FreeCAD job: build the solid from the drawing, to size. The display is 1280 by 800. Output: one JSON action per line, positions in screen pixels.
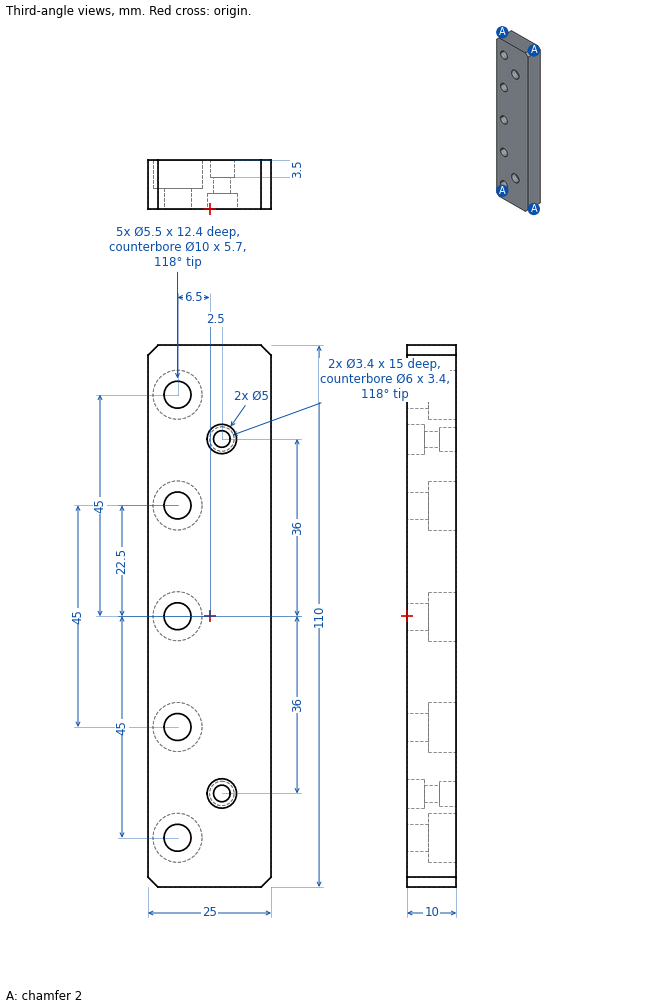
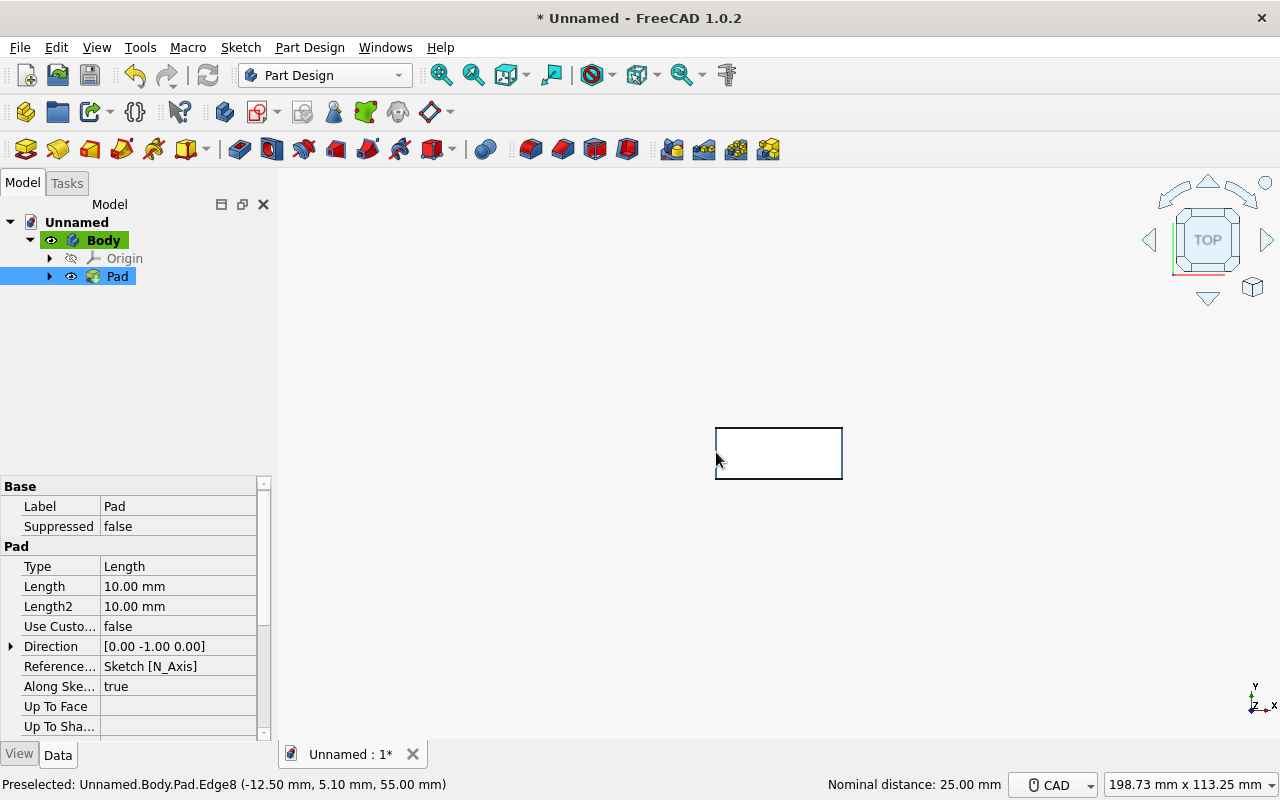
{"action": "key", "text": "1"}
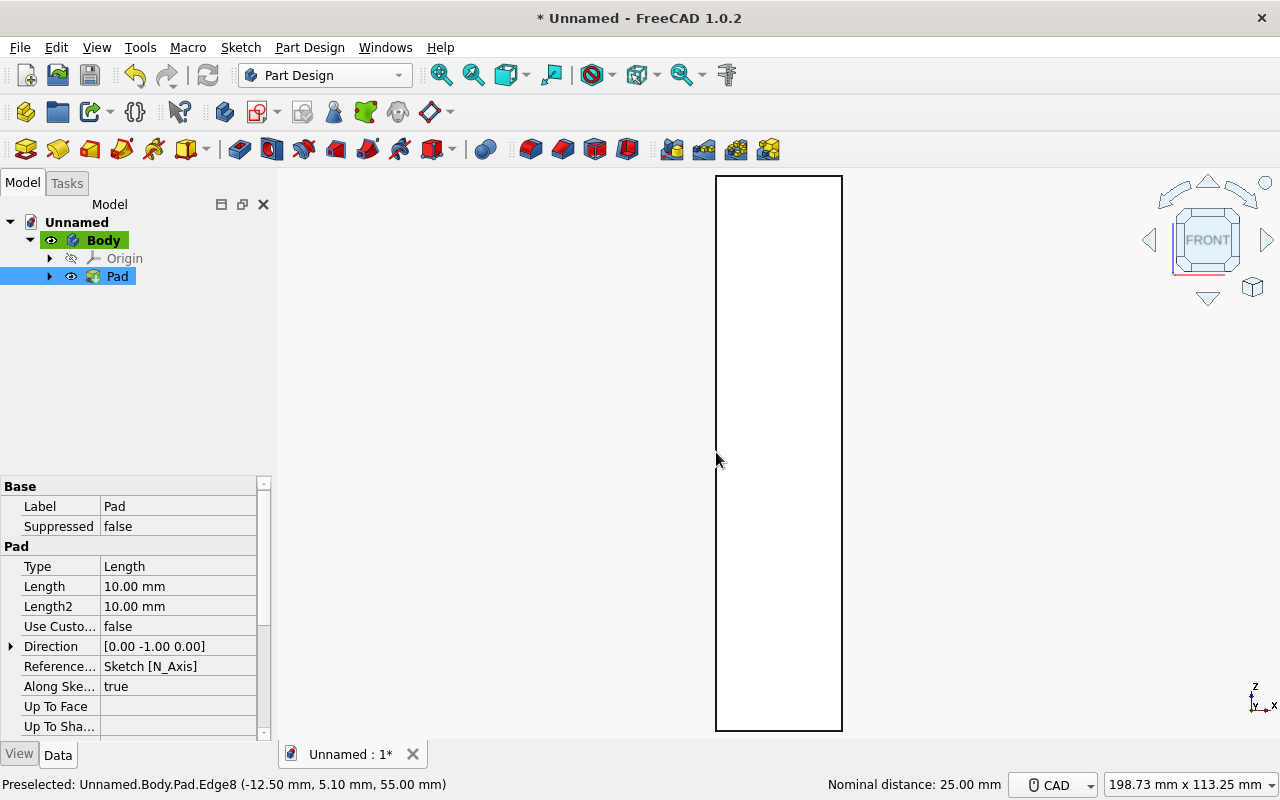
{"action": "key", "text": "3"}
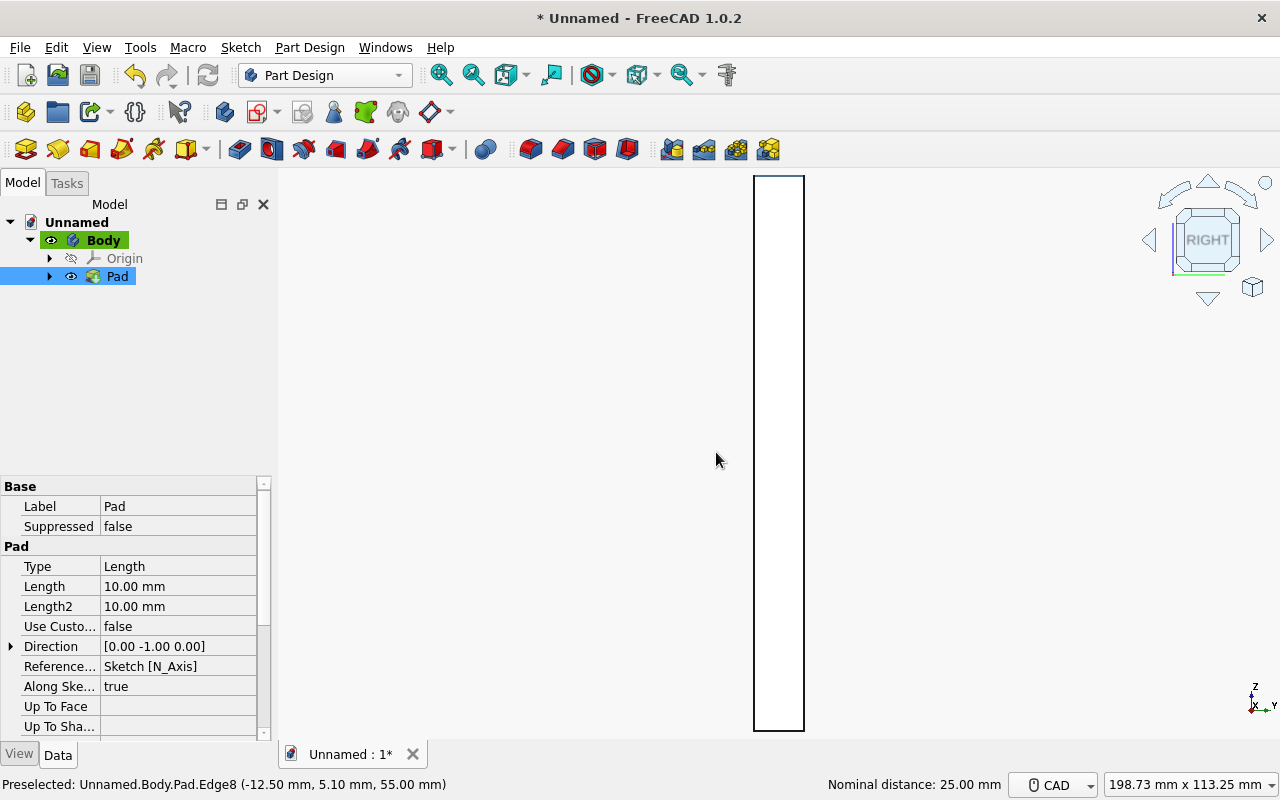
{"action": "key", "text": "5"}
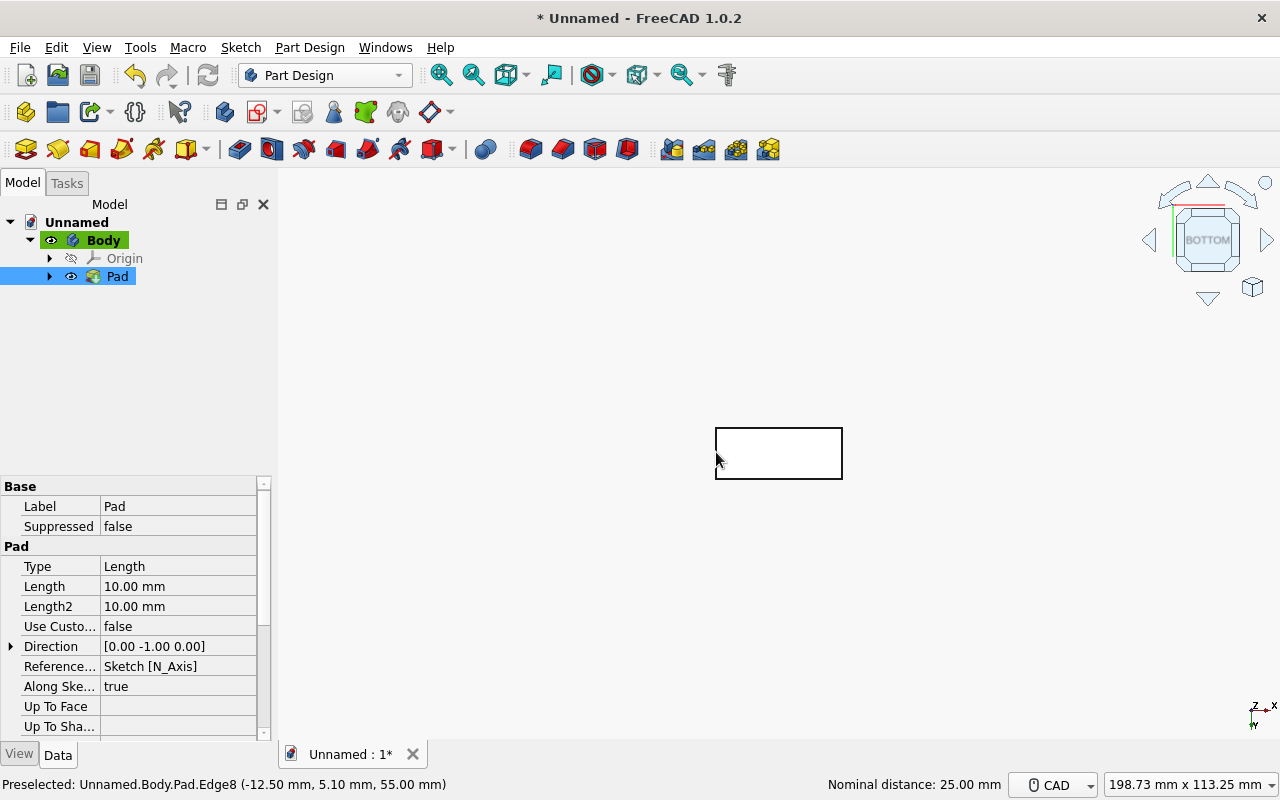
{"action": "left_click", "coordinate": [442, 76]}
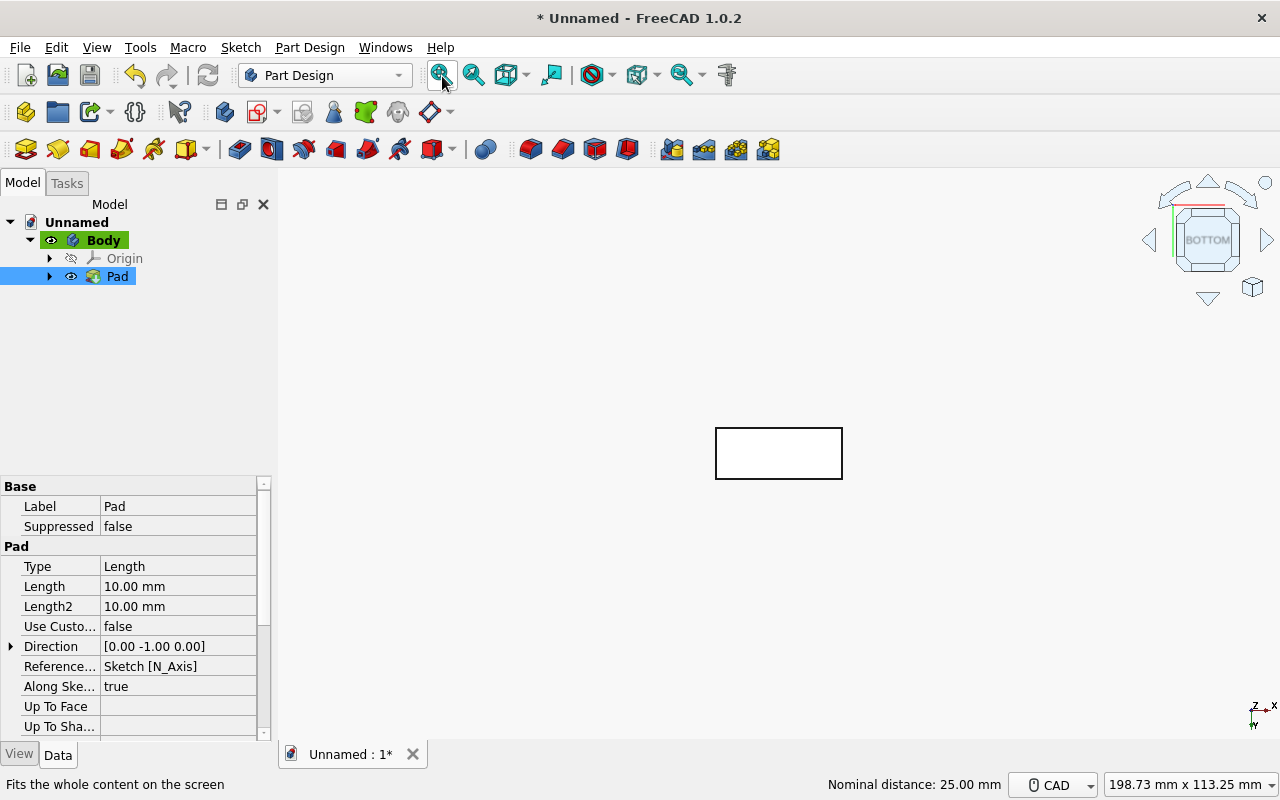
{"action": "left_click", "coordinate": [716, 452], "text": "ctrl"}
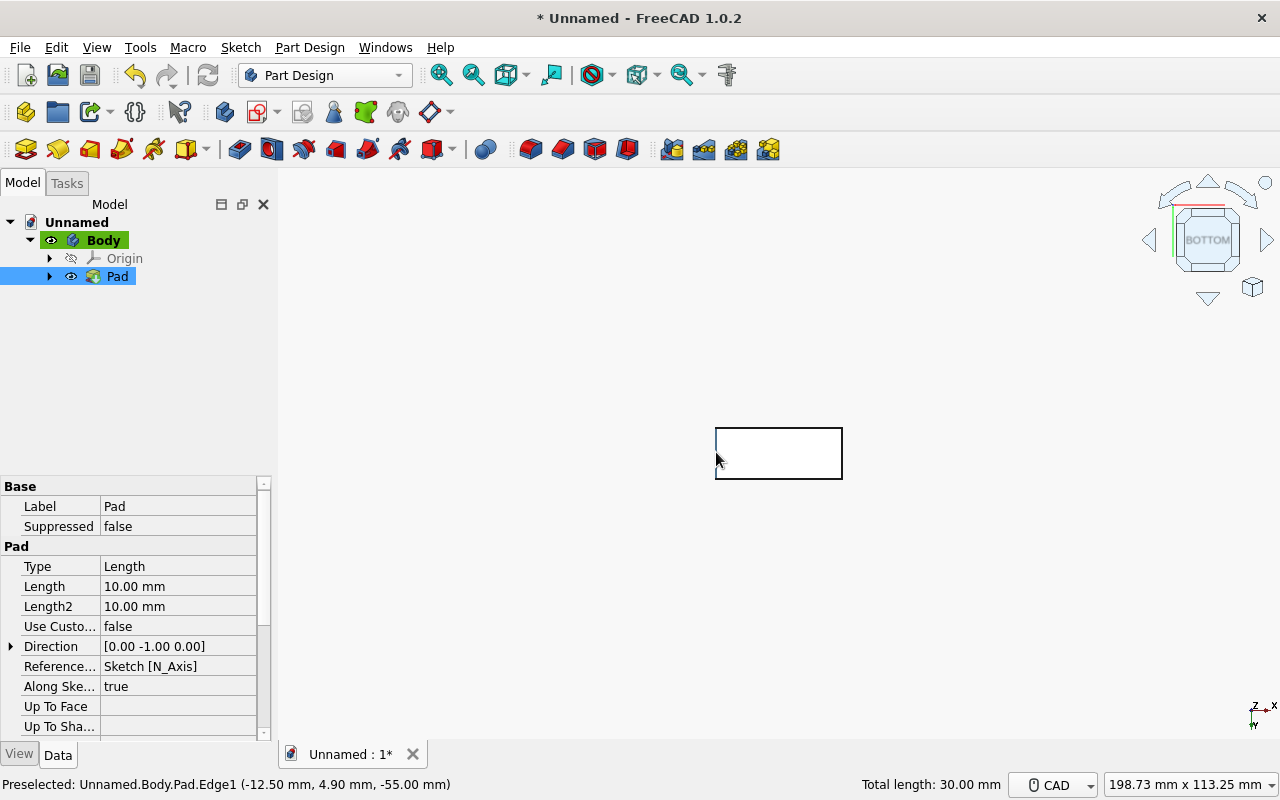
{"action": "left_click", "coordinate": [842, 452], "text": "ctrl"}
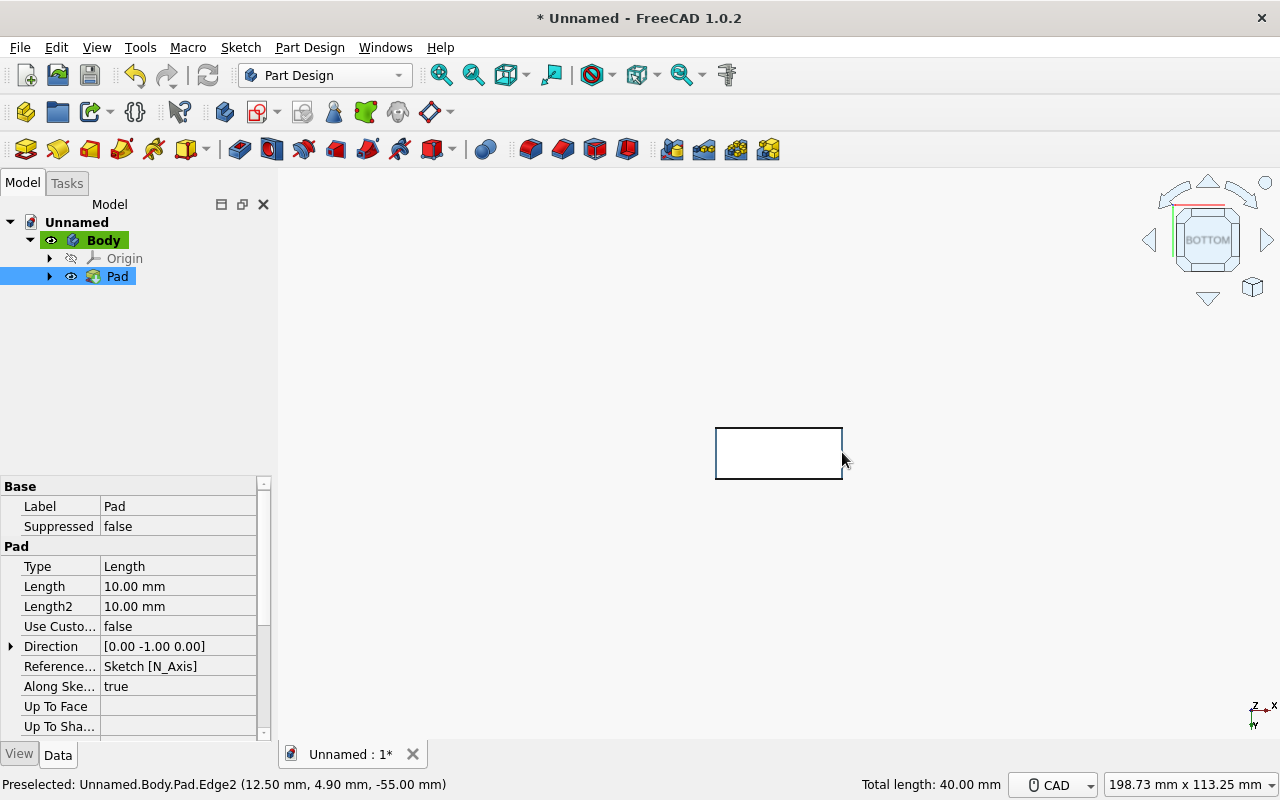
{"action": "left_click", "coordinate": [564, 150]}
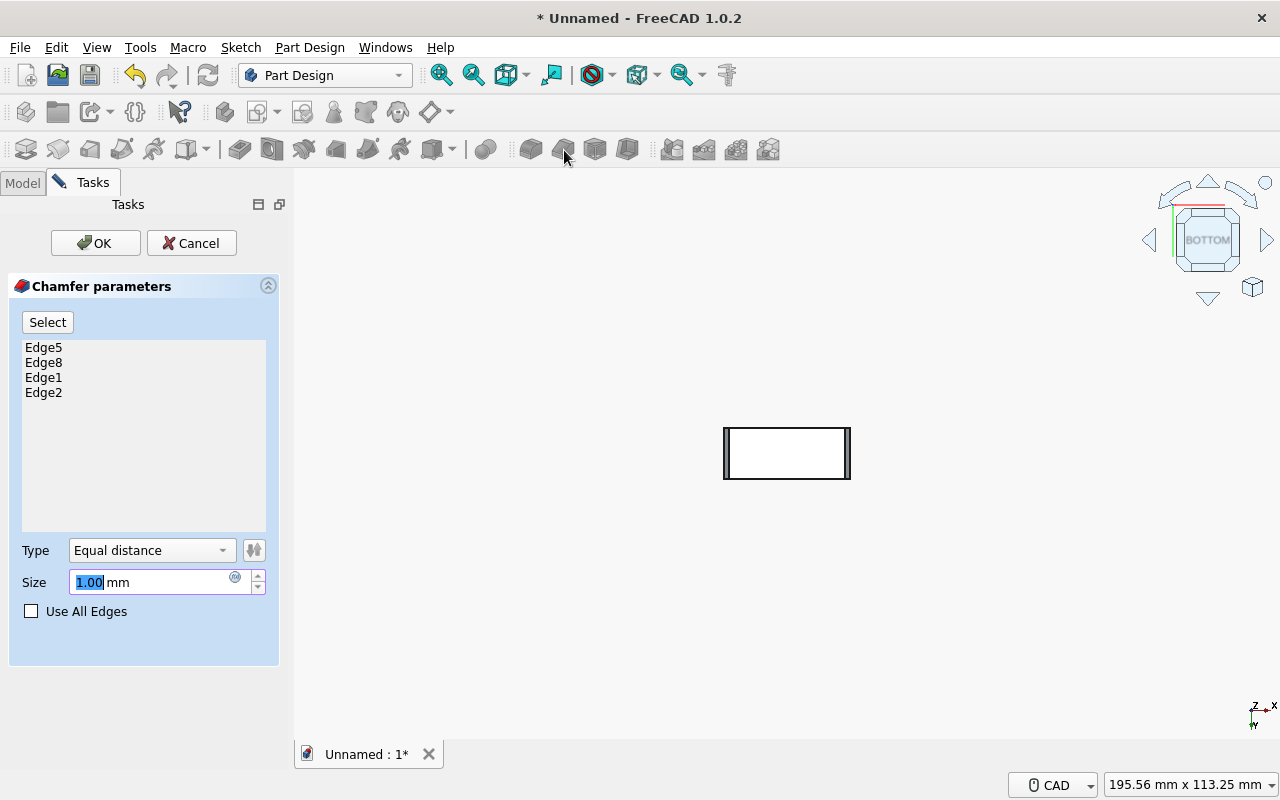
{"action": "type", "text": "2"}
{"action": "key", "text": "Tab"}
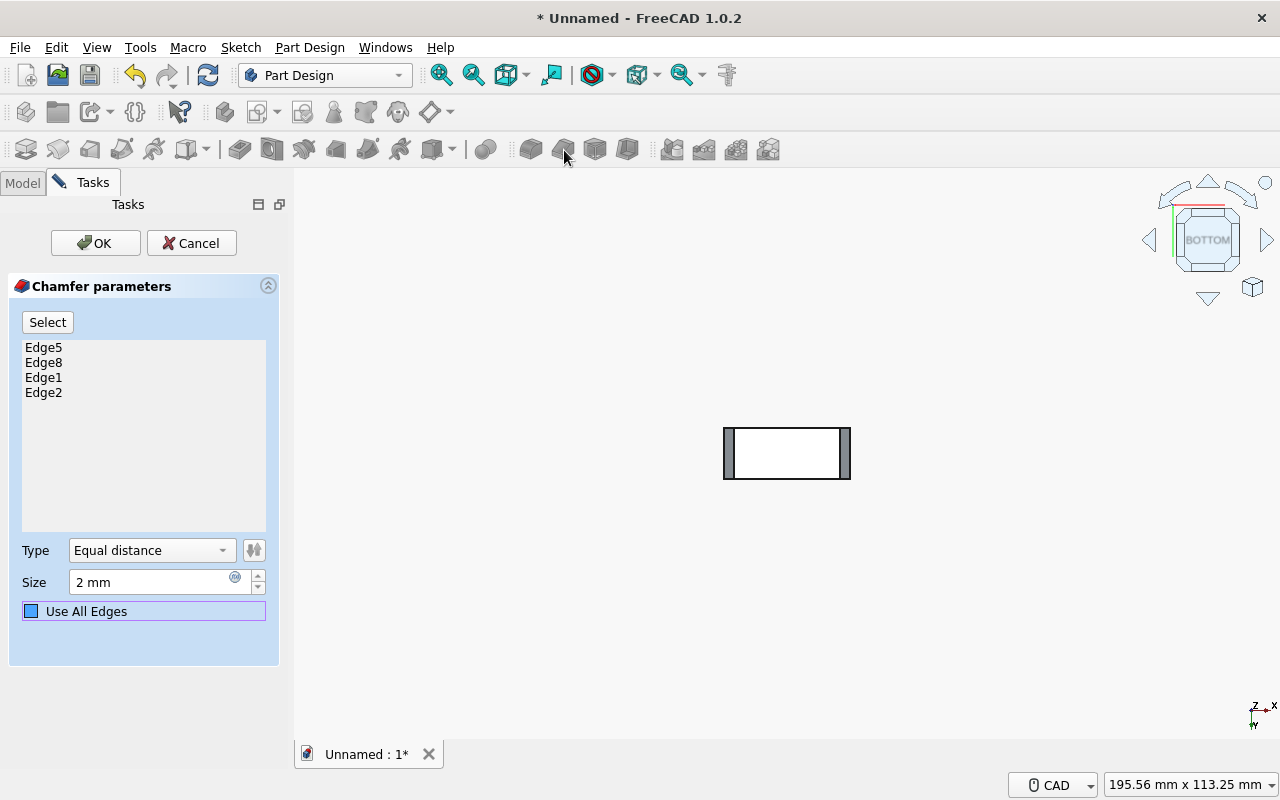
{"action": "left_click", "coordinate": [96, 243]}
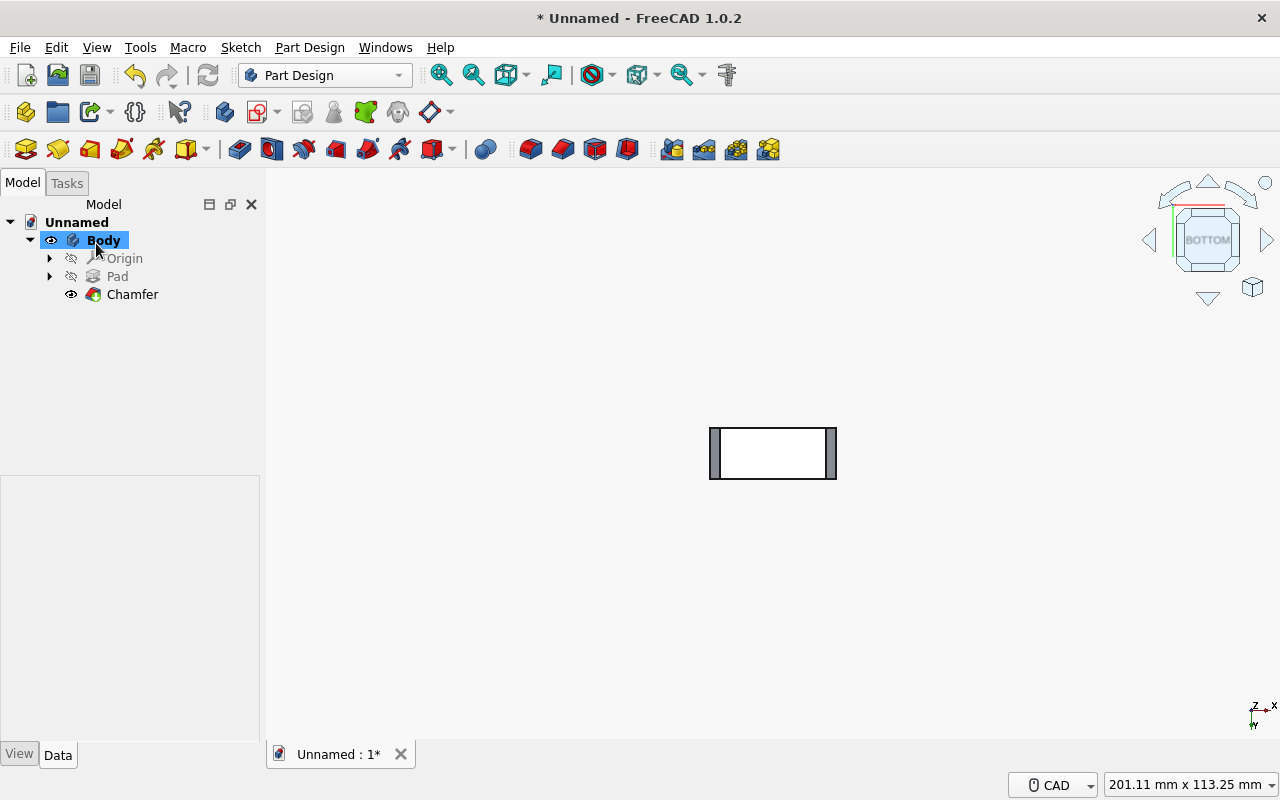
{"action": "left_click", "coordinate": [442, 76]}